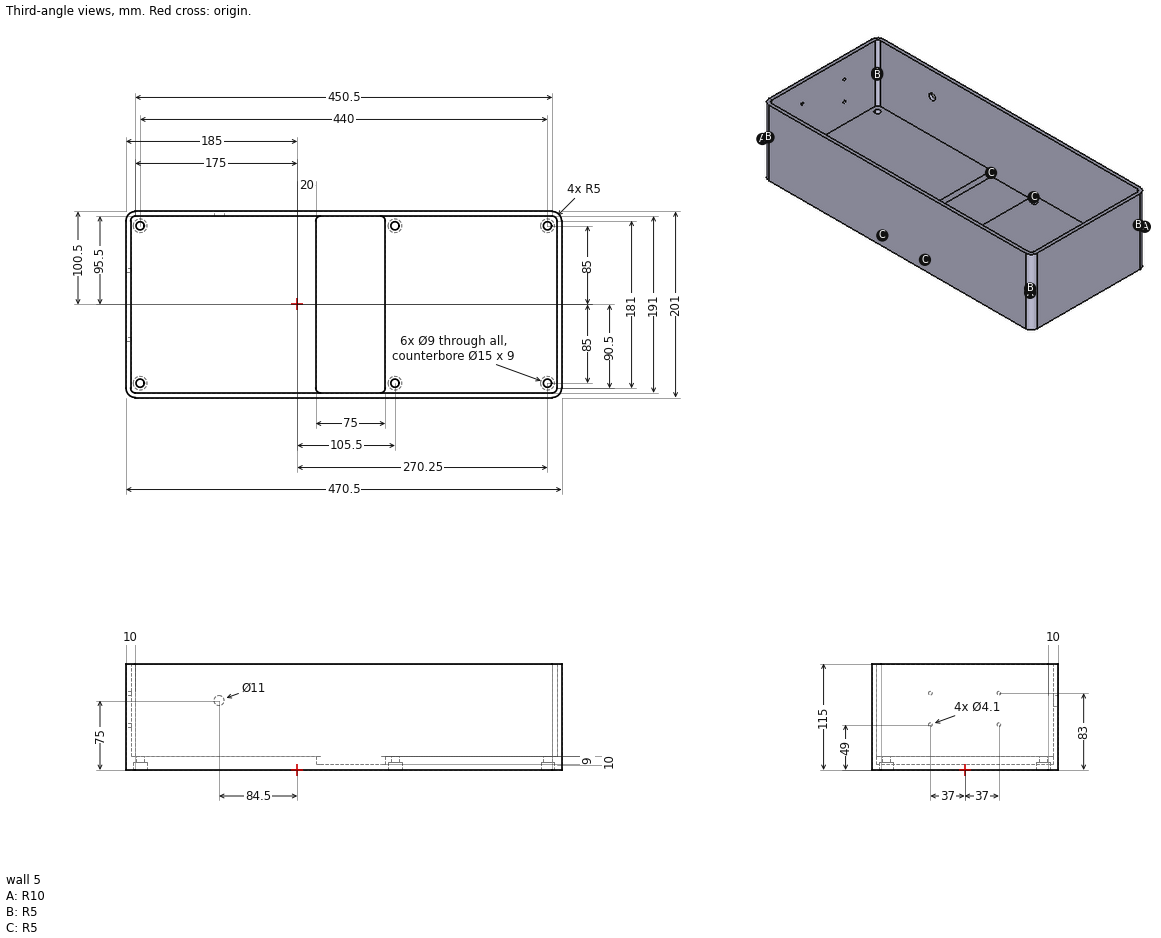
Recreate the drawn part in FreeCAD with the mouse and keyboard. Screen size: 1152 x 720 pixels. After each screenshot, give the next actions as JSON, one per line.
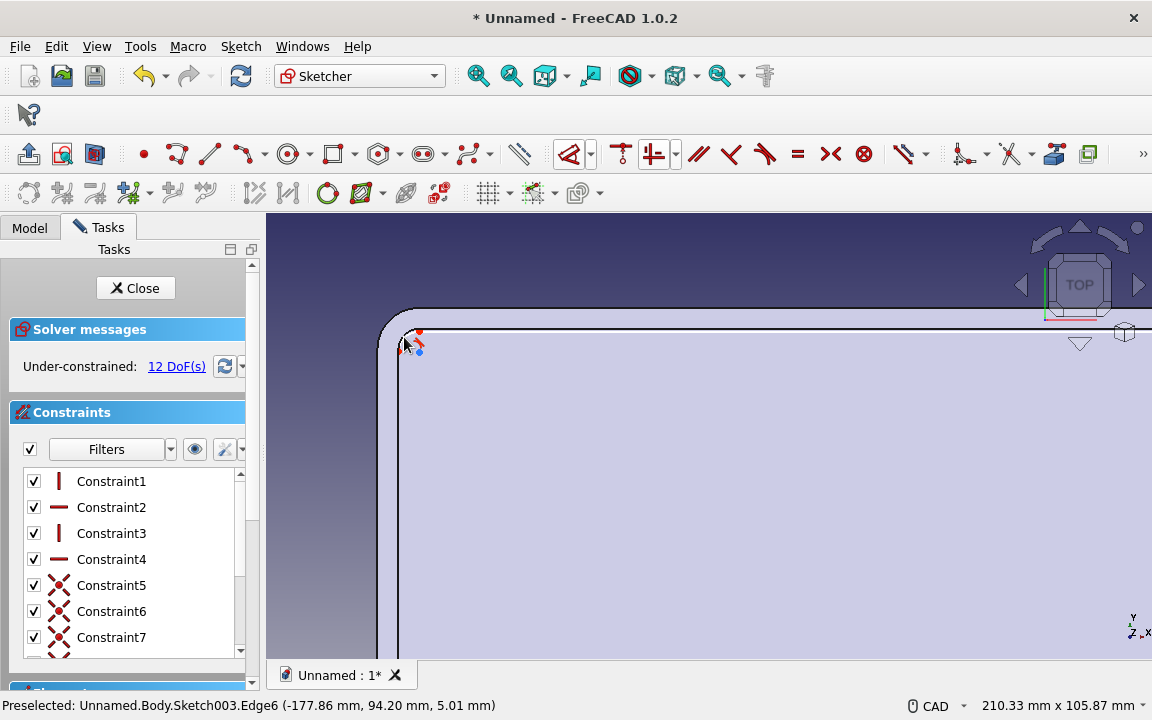
{"action": "scroll", "coordinate": [402, 339], "scroll_direction": "down", "scroll_amount": 7}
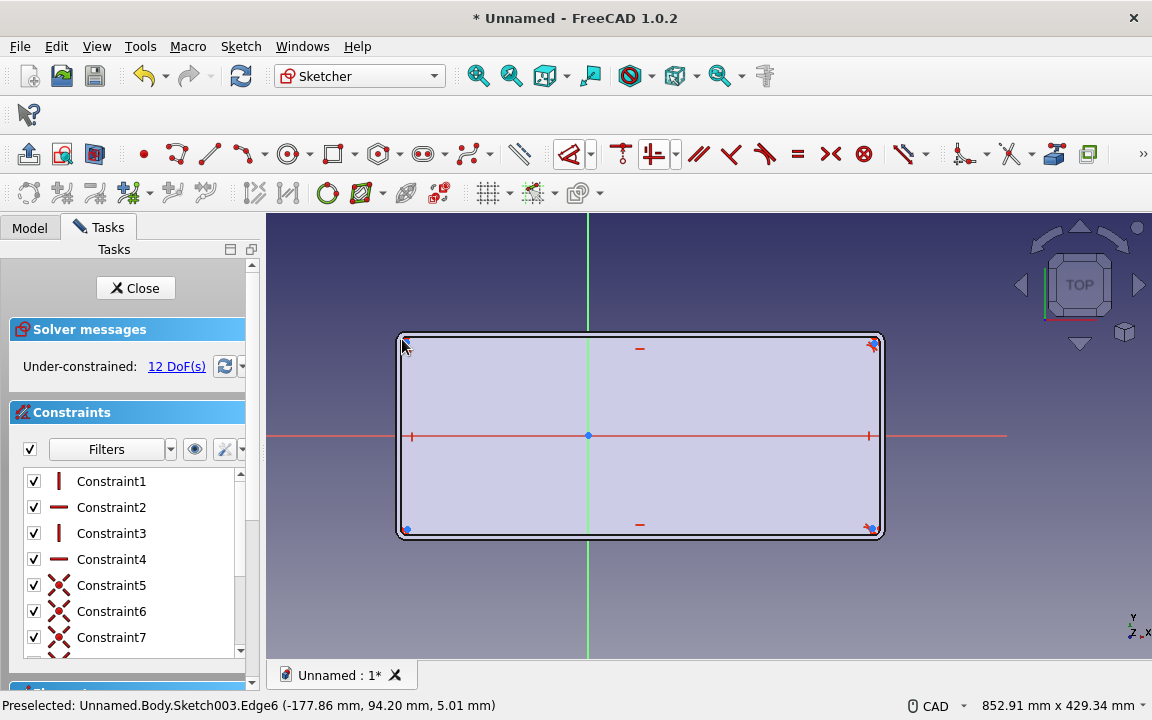
{"action": "left_click", "coordinate": [401, 399]}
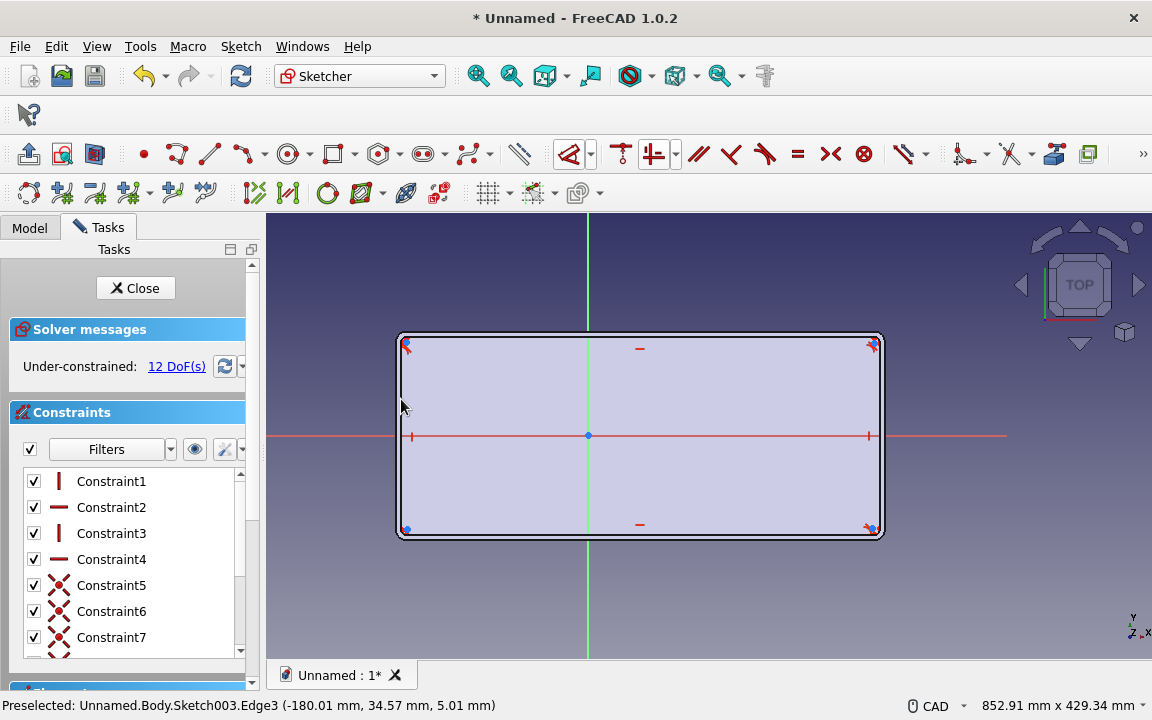
{"action": "scroll", "coordinate": [403, 339], "scroll_direction": "up", "scroll_amount": 7}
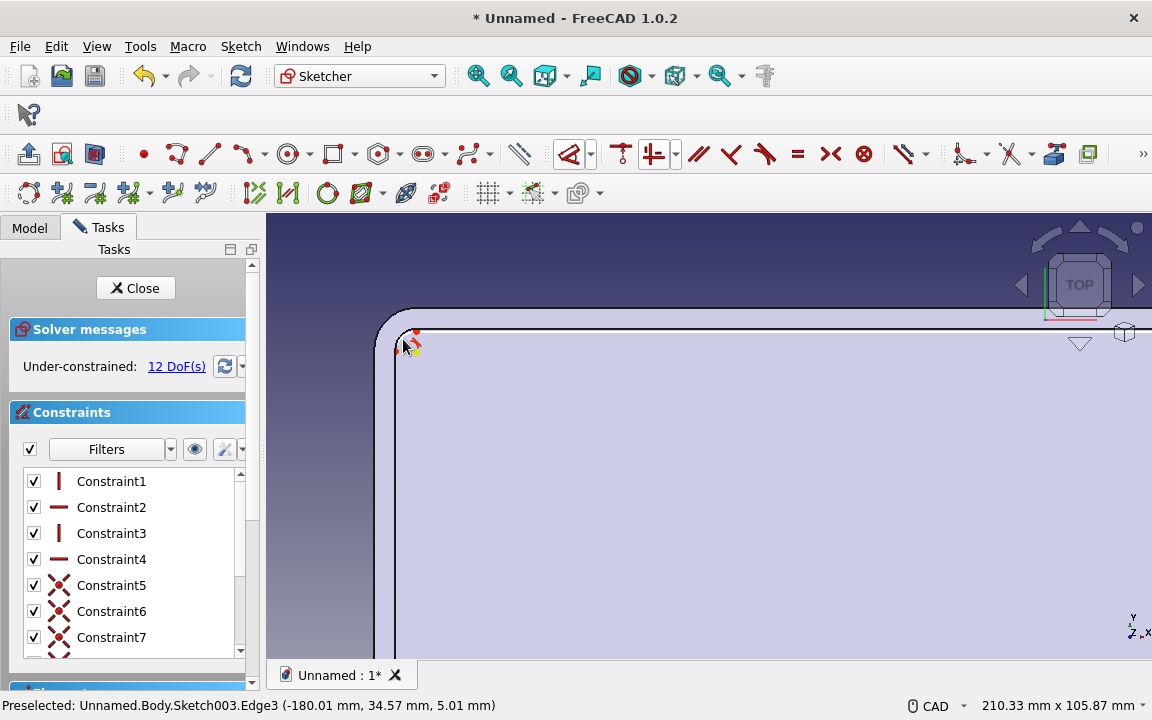
{"action": "left_click", "coordinate": [402, 338]}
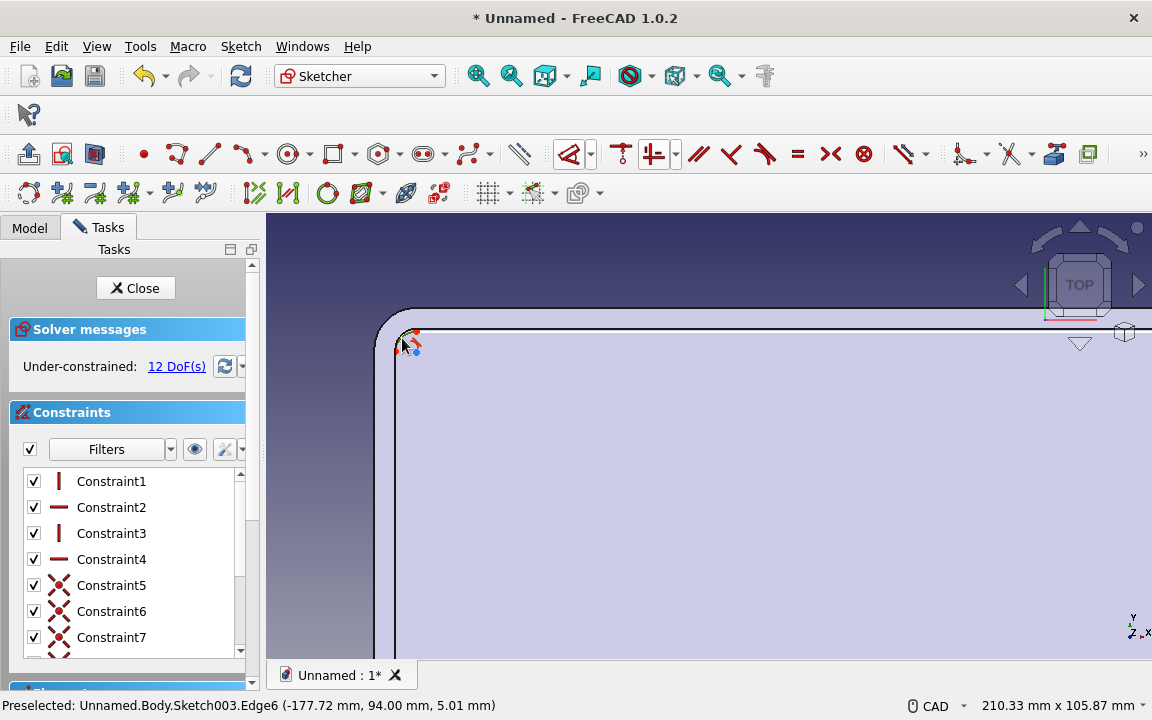
{"action": "key", "text": "t"}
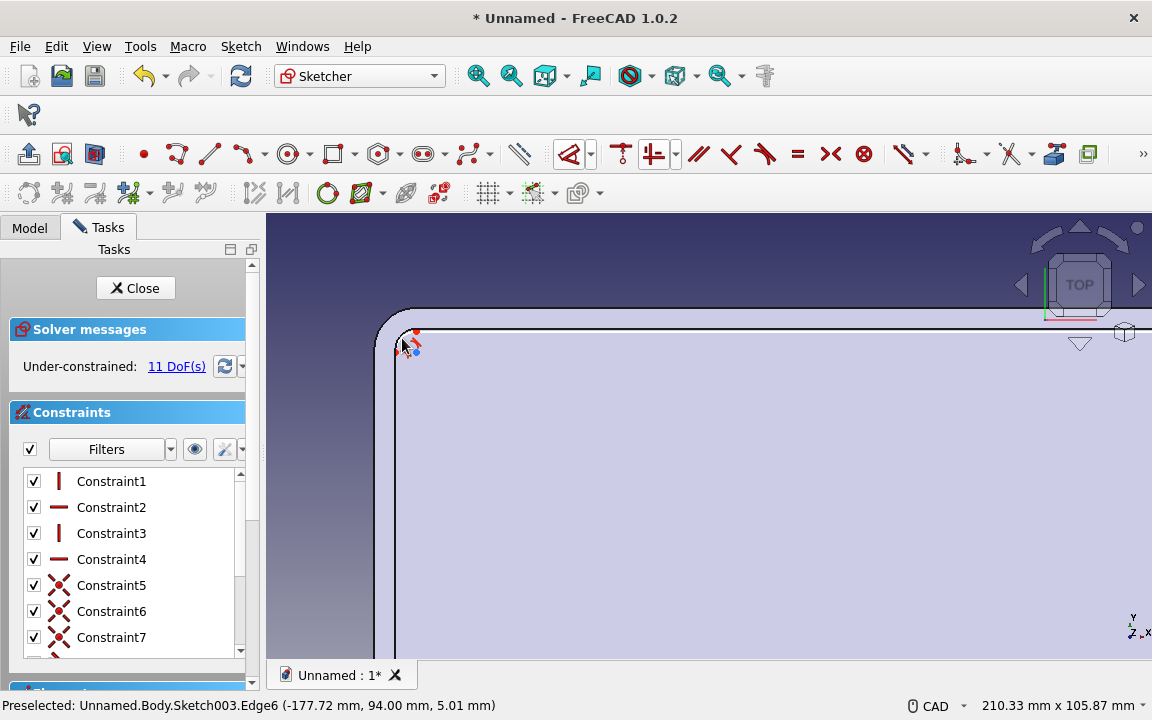
{"action": "scroll", "coordinate": [403, 339], "scroll_direction": "down", "scroll_amount": 7}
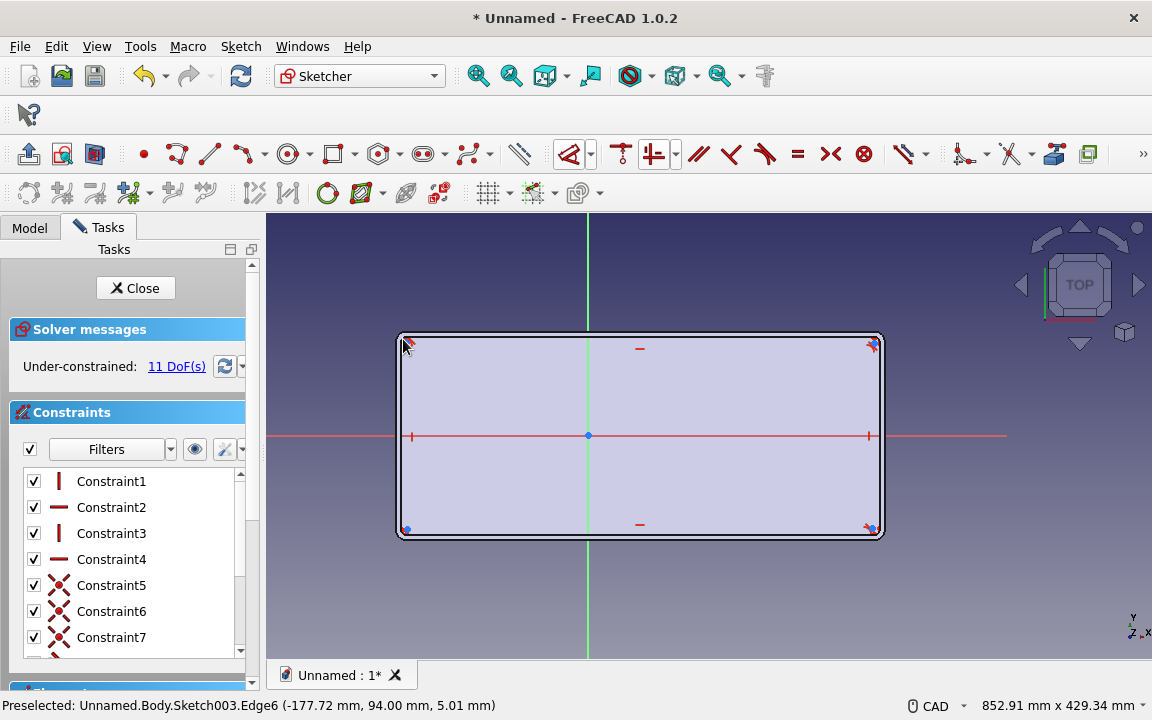
{"action": "left_click", "coordinate": [401, 399]}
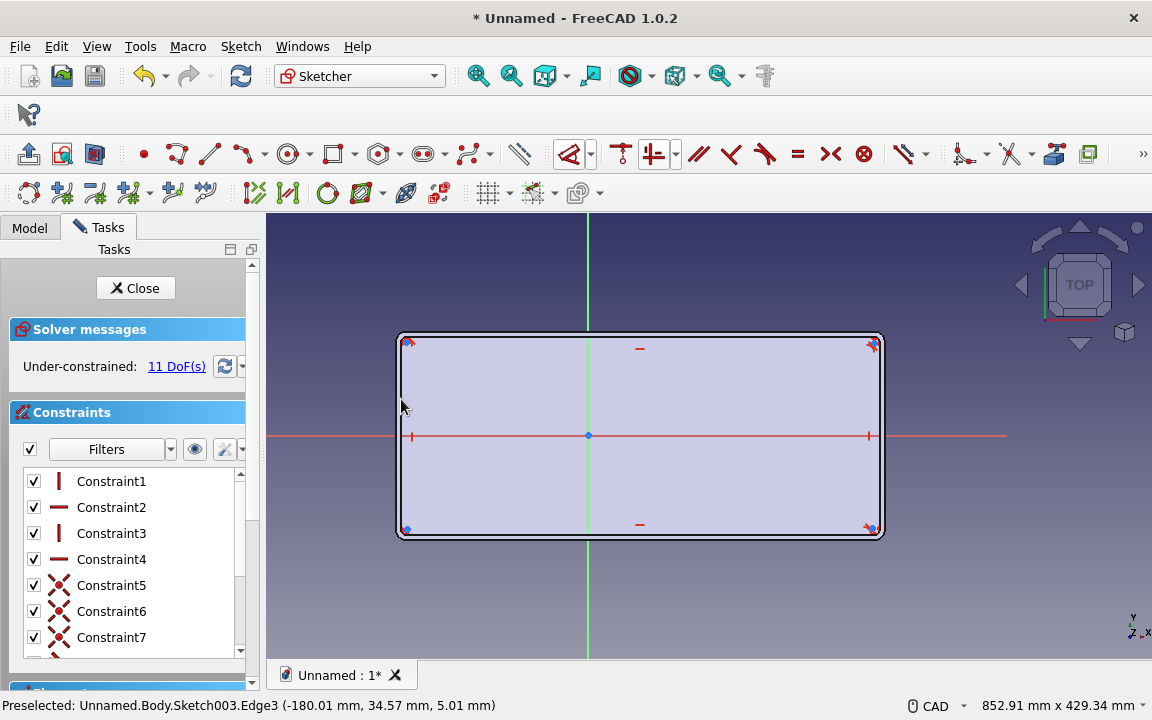
{"action": "scroll", "coordinate": [403, 534], "scroll_direction": "up", "scroll_amount": 7}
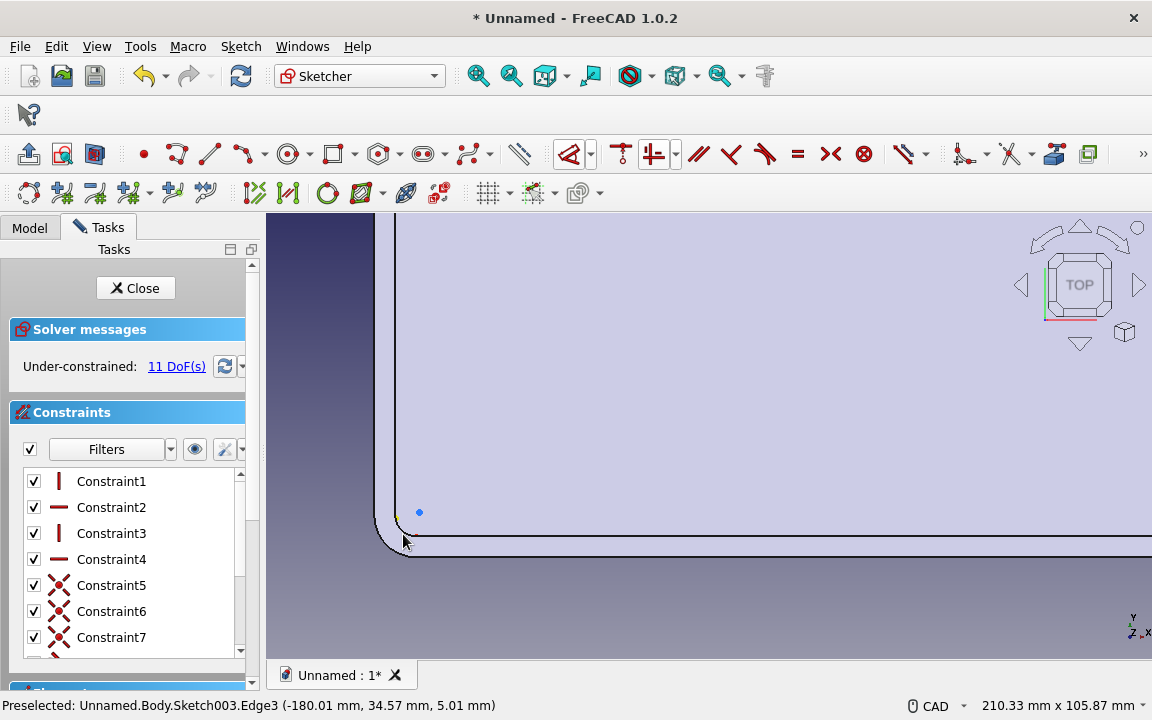
{"action": "left_click", "coordinate": [403, 531]}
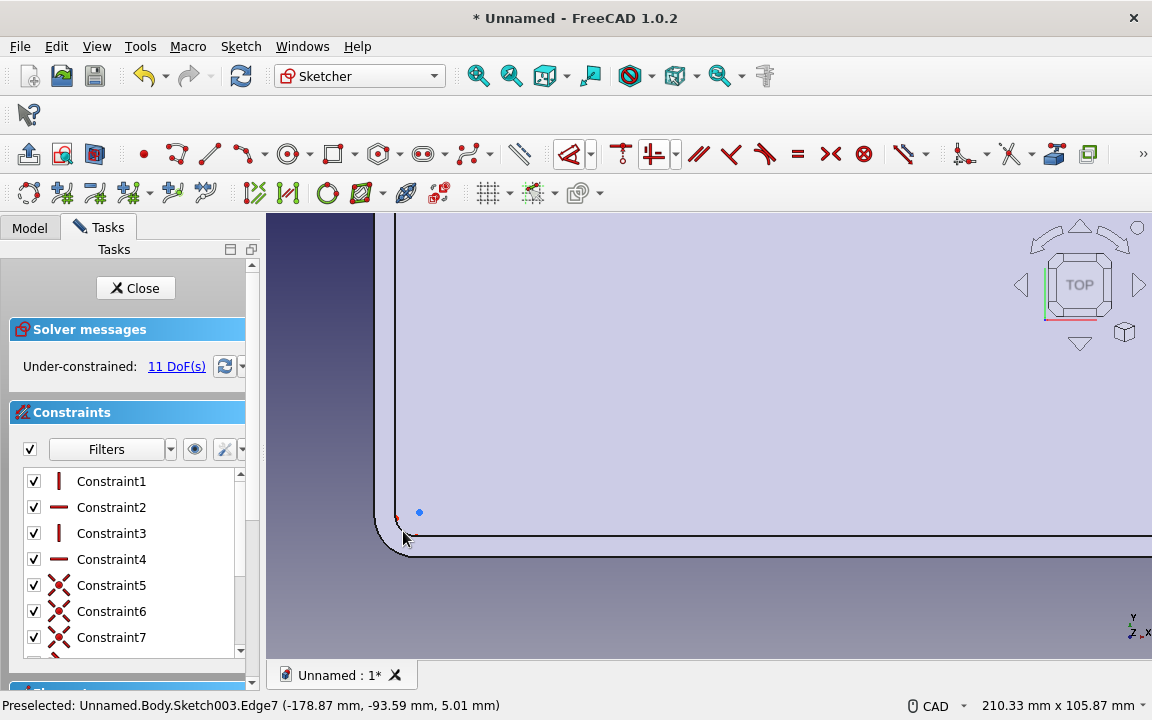
{"action": "key", "text": "t"}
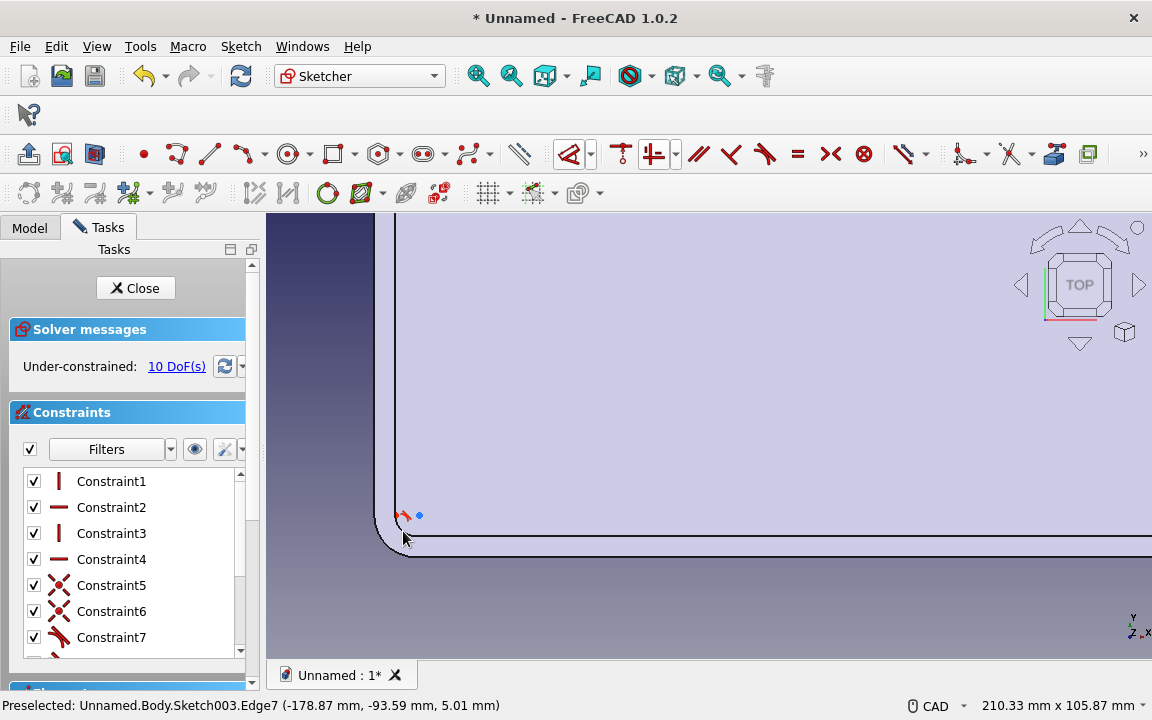
{"action": "scroll", "coordinate": [403, 535], "scroll_direction": "down", "scroll_amount": 7}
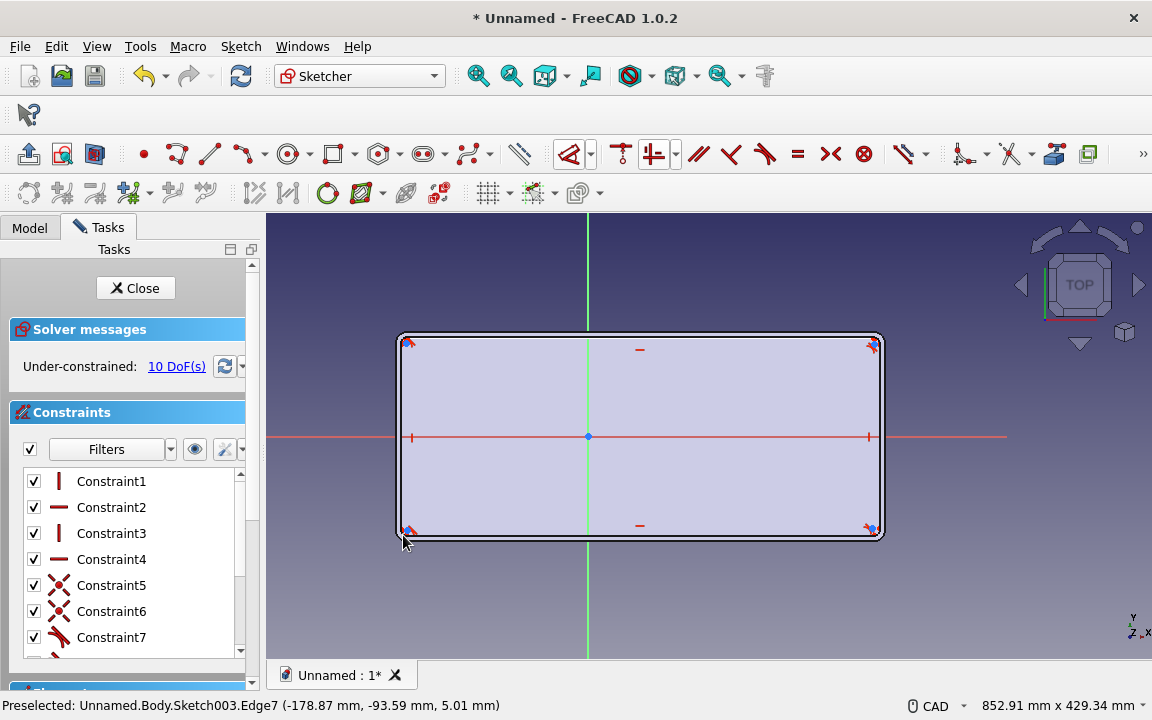
{"action": "left_click", "coordinate": [547, 537]}